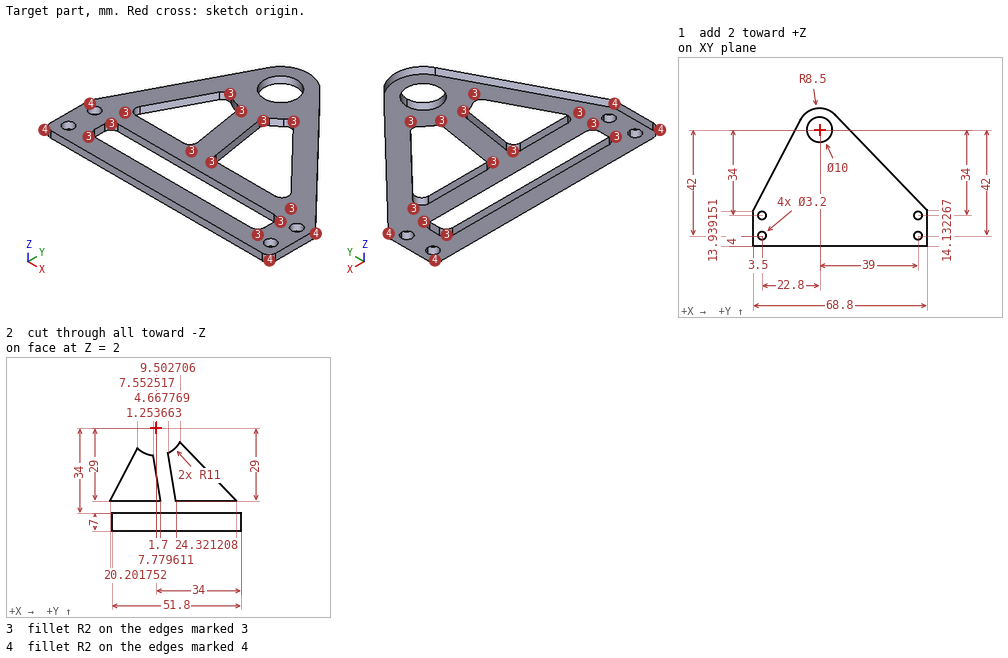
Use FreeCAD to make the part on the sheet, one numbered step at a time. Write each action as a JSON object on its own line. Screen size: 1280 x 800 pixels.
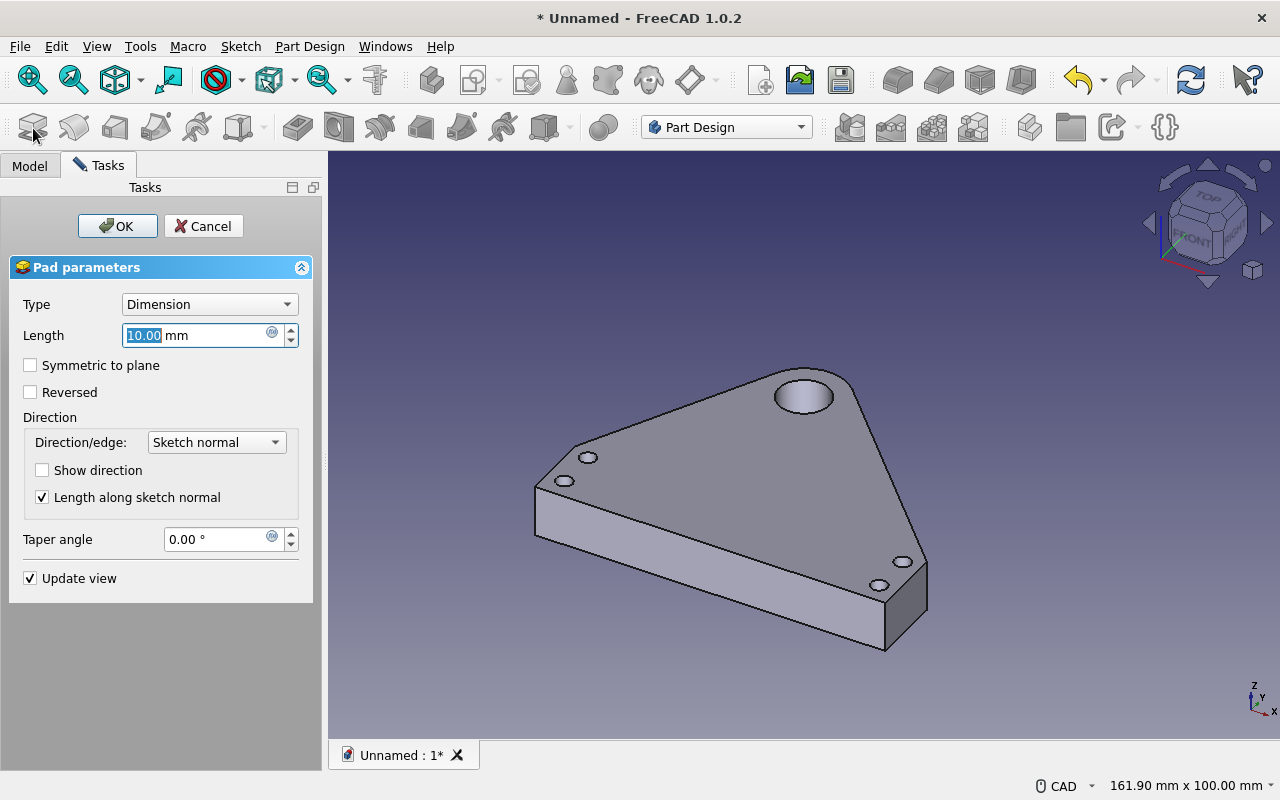
{"action": "type", "text": "2"}
{"action": "key", "text": "Tab"}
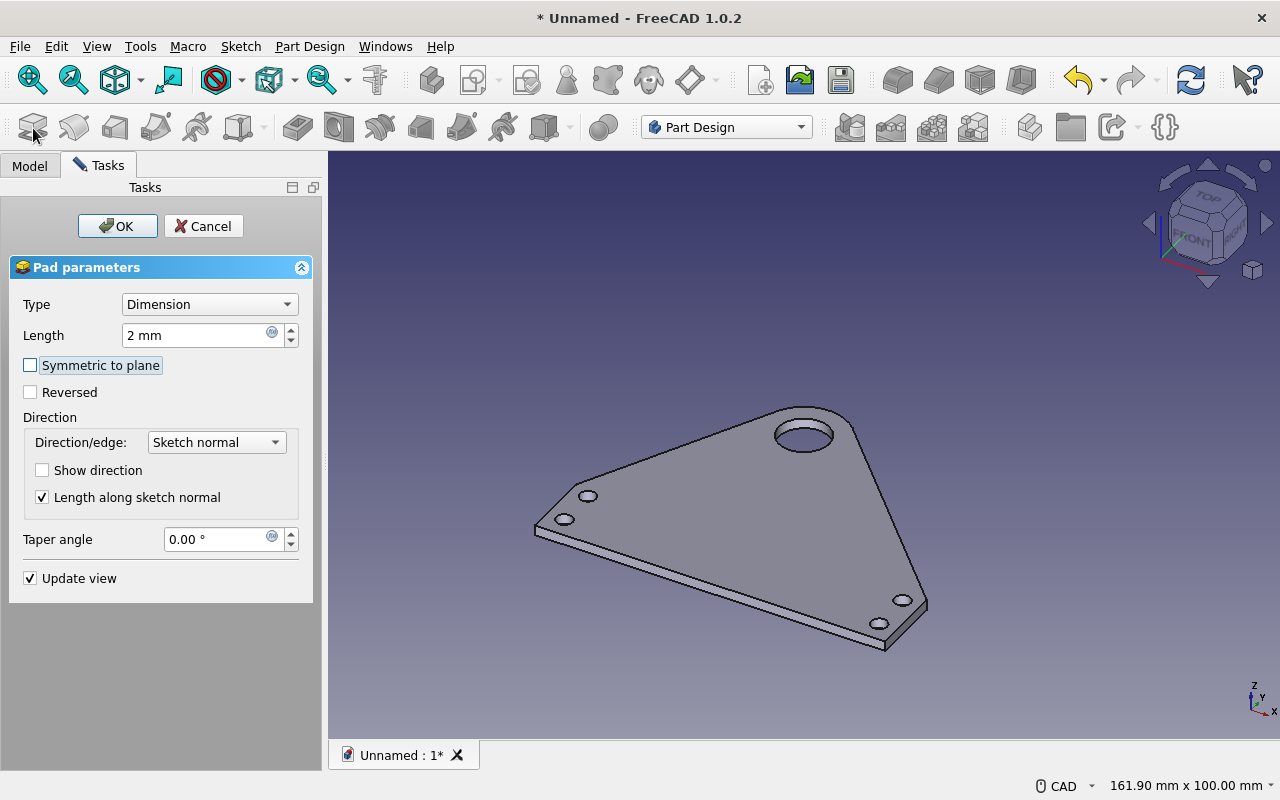
{"action": "left_click", "coordinate": [118, 226]}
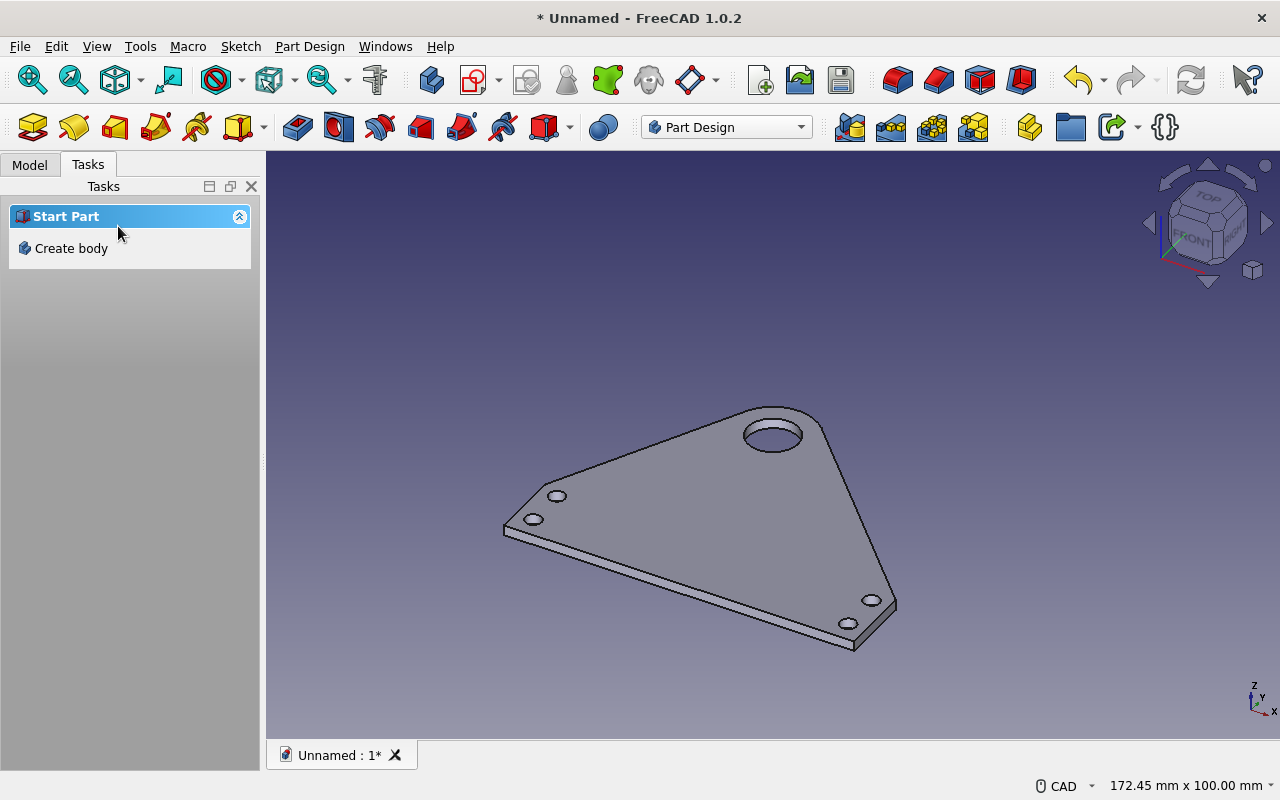
{"action": "left_click", "coordinate": [736, 526]}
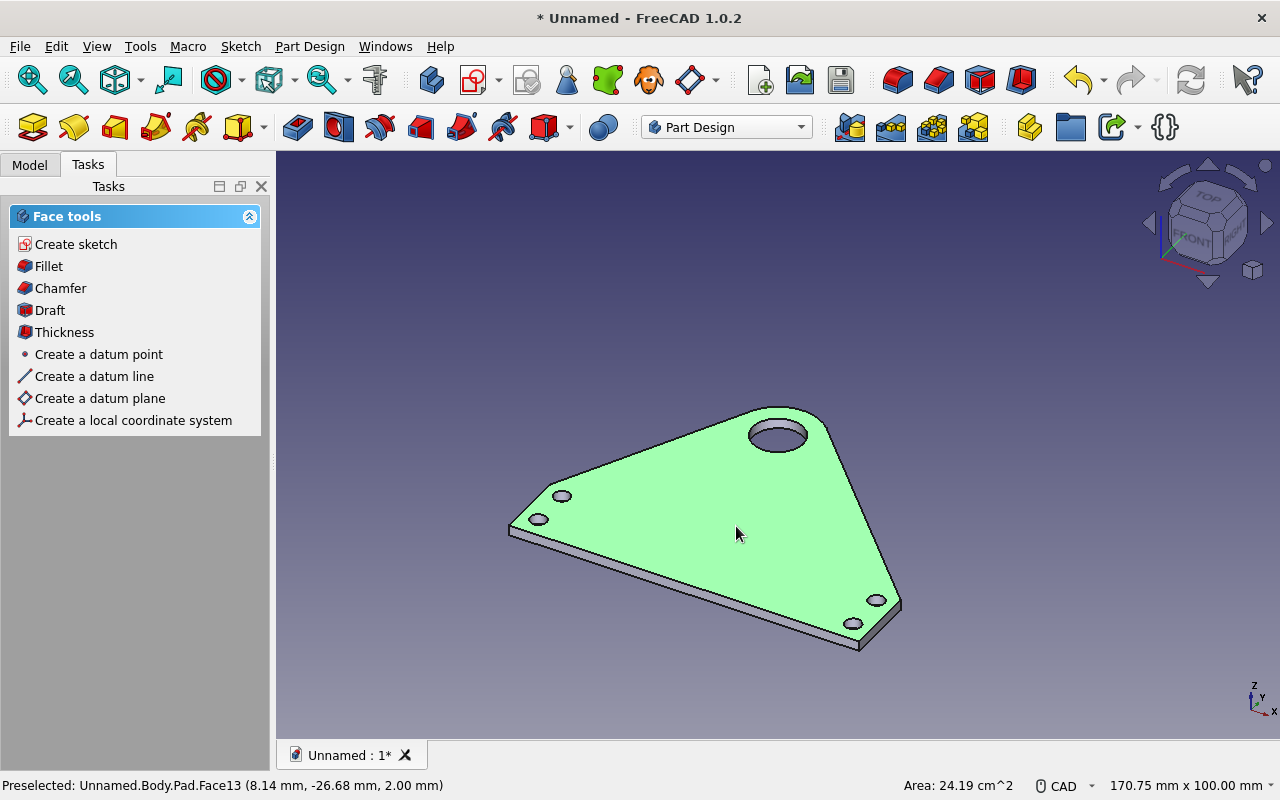
{"action": "left_click", "coordinate": [472, 80]}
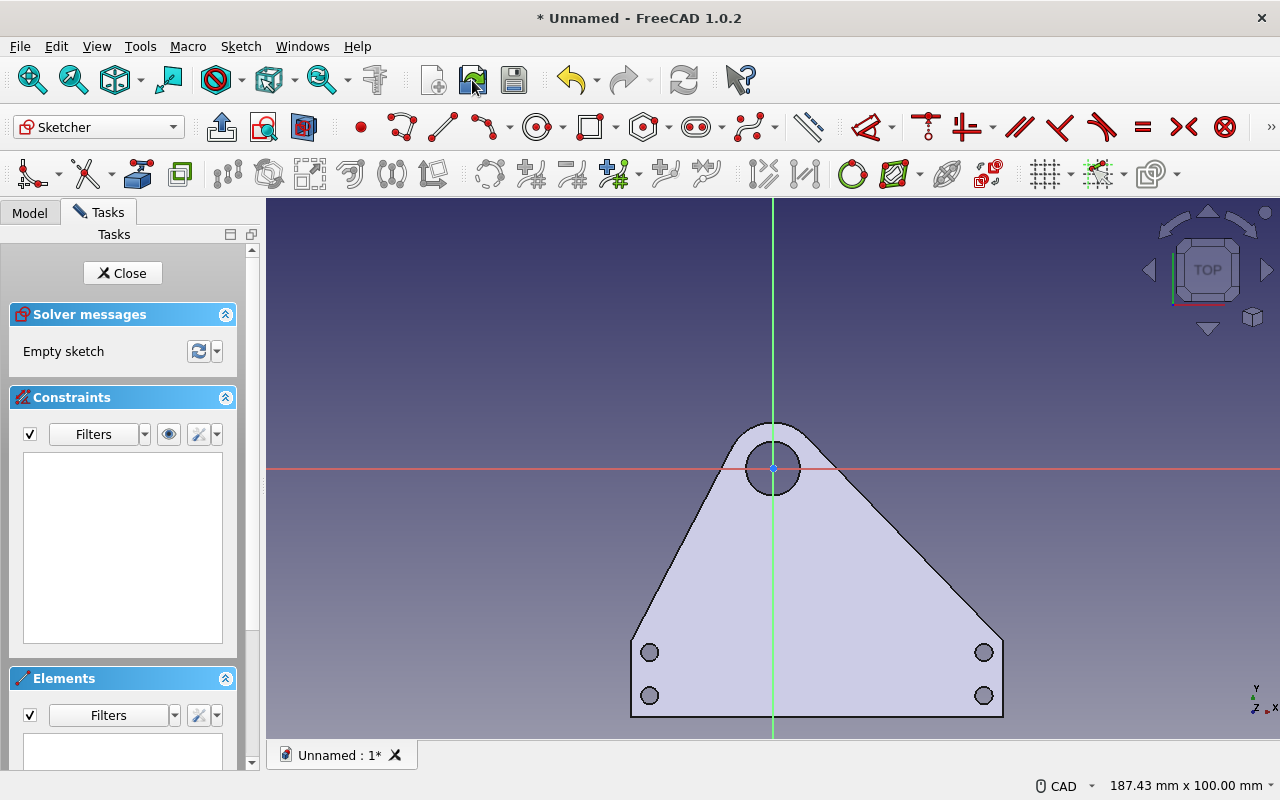
{"action": "scroll", "coordinate": [1039, 711], "scroll_direction": "up", "scroll_amount": 2}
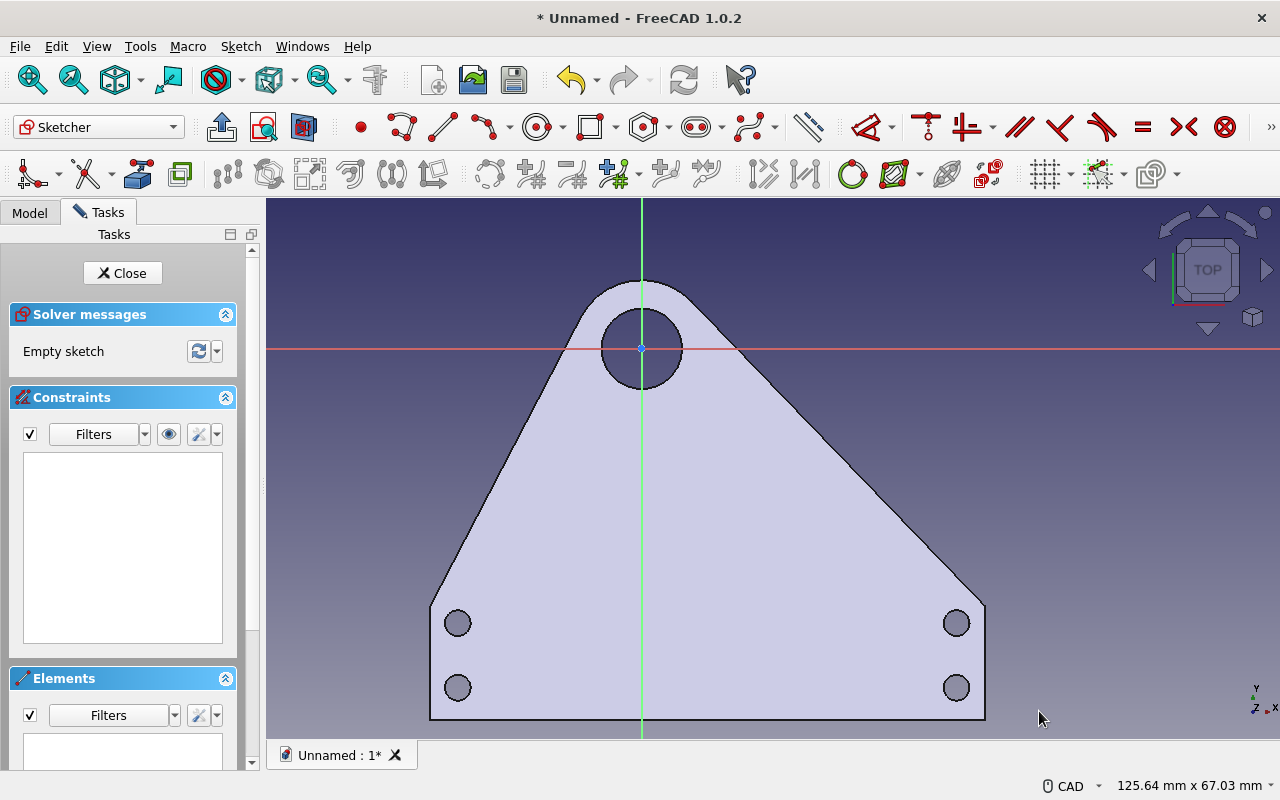
{"action": "key", "text": "g m"}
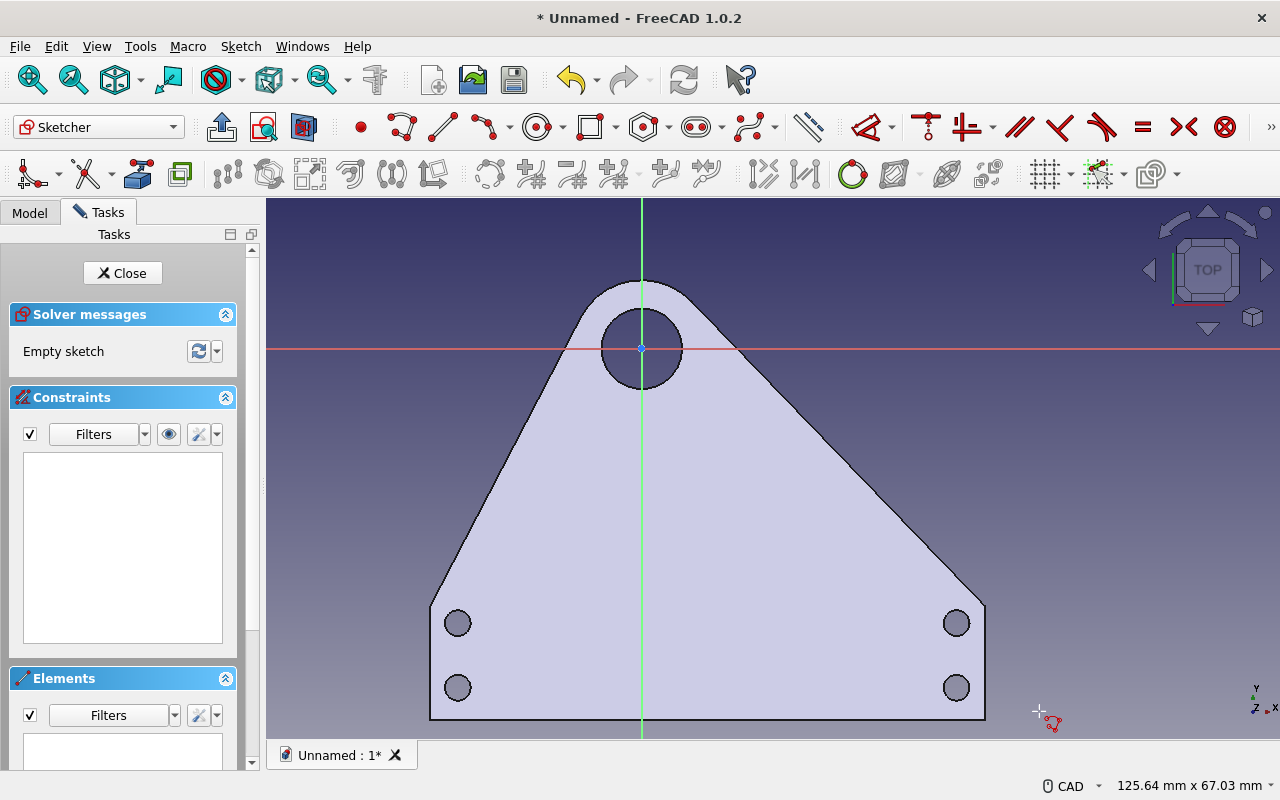
{"action": "left_click", "coordinate": [581, 413]}
{"action": "left_click", "coordinate": [492, 583]}
{"action": "left_click", "coordinate": [656, 583]}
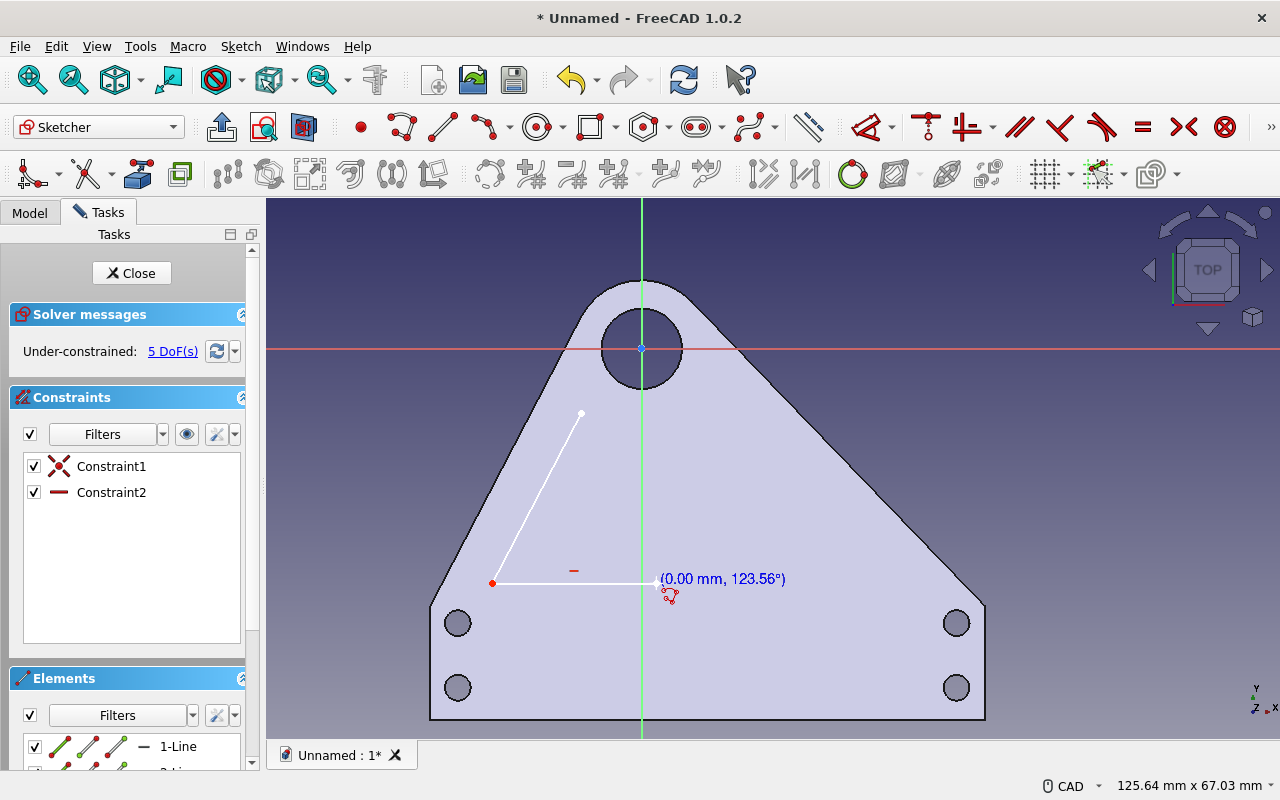
{"action": "scroll", "coordinate": [632, 437], "scroll_direction": "up", "scroll_amount": 3}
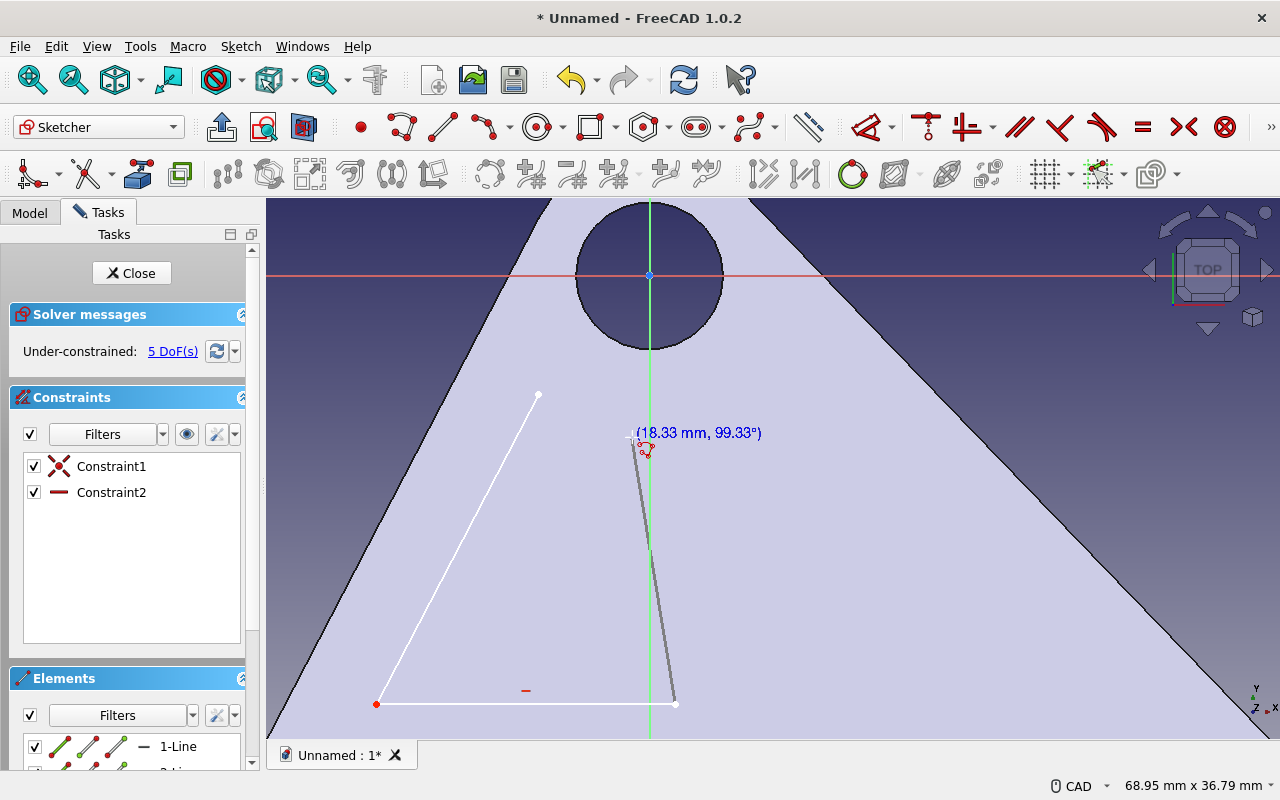
{"action": "left_click", "coordinate": [631, 437]}
{"action": "right_click", "coordinate": [631, 437]}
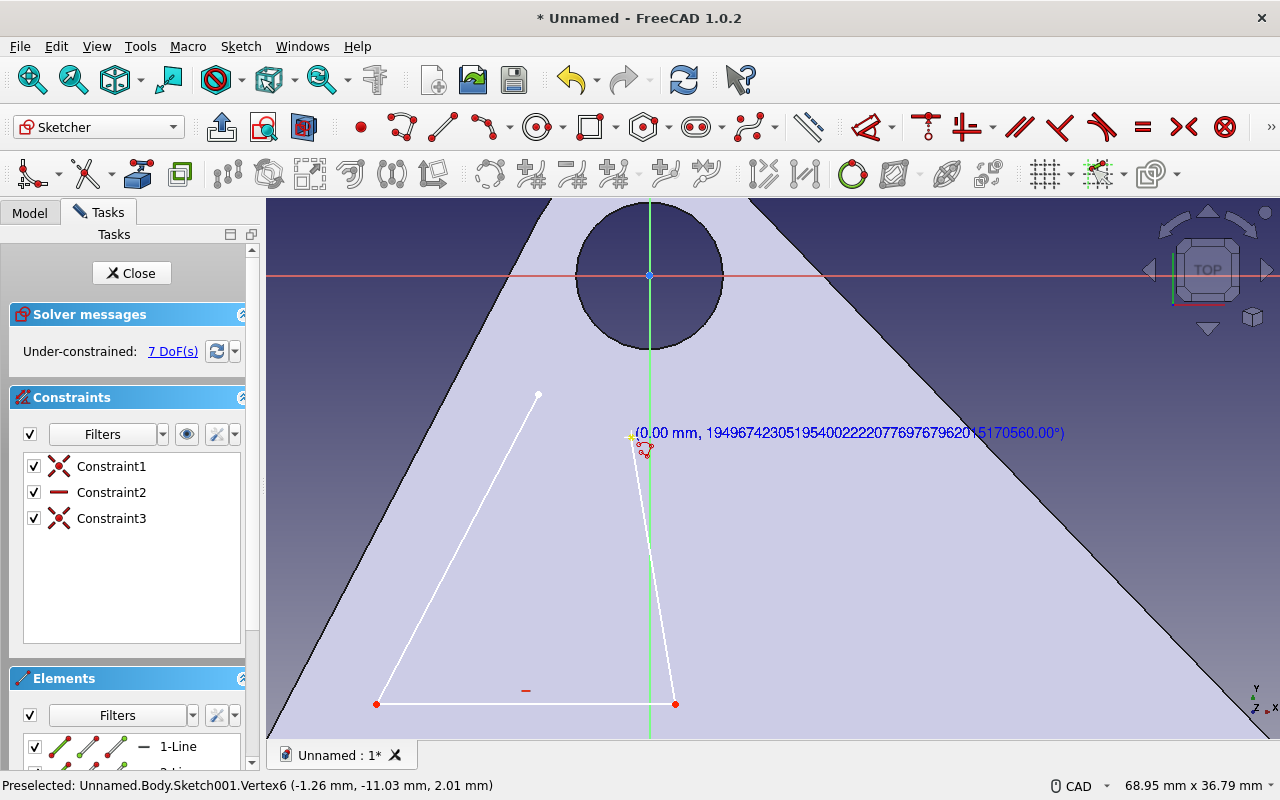
{"action": "left_click", "coordinate": [484, 128]}